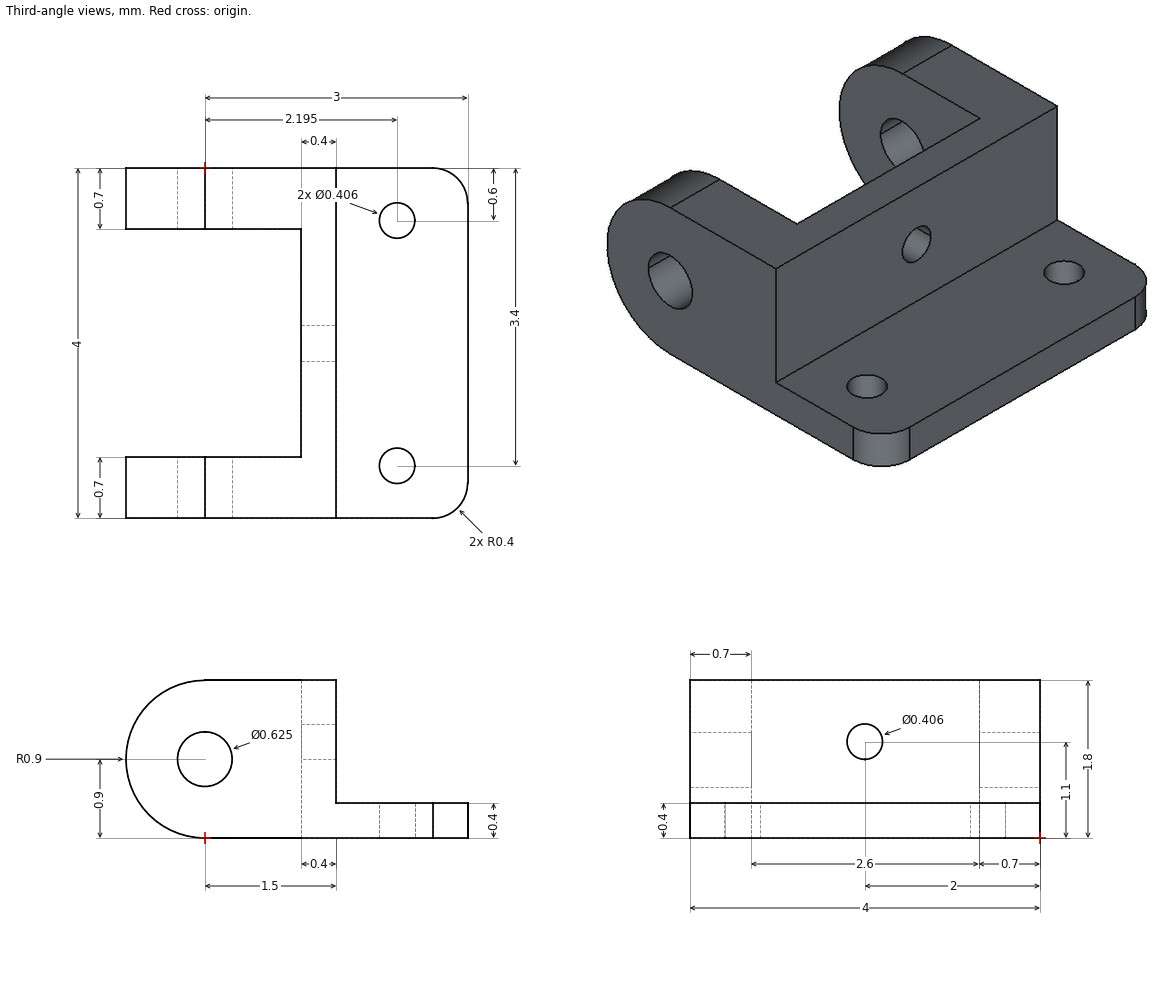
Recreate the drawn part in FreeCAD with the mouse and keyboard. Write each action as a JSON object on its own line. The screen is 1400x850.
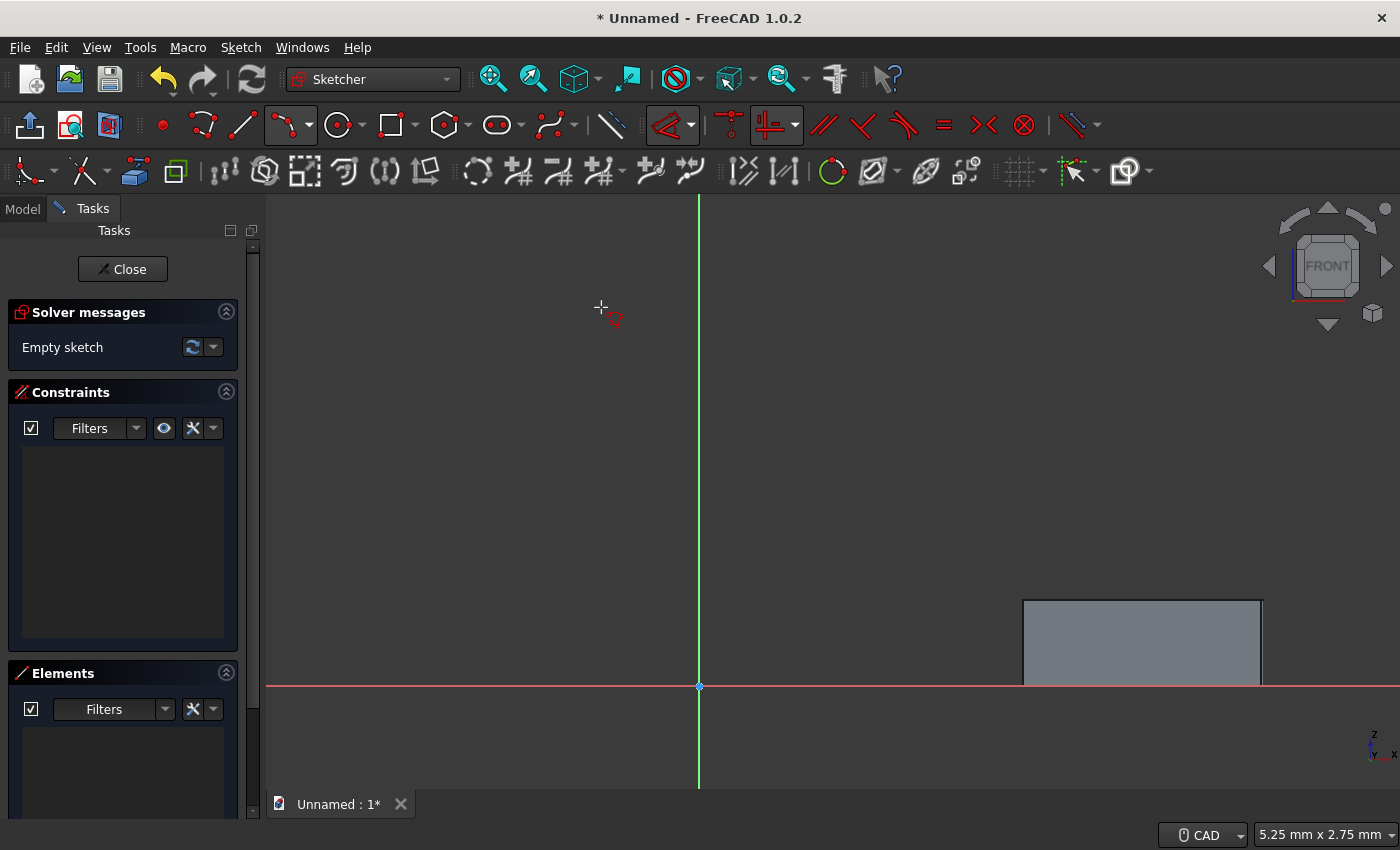
{"action": "left_click", "coordinate": [699, 297]}
{"action": "left_click", "coordinate": [1023, 297]}
{"action": "left_click", "coordinate": [1023, 686]}
{"action": "left_click", "coordinate": [699, 686]}
{"action": "right_click", "coordinate": [699, 686]}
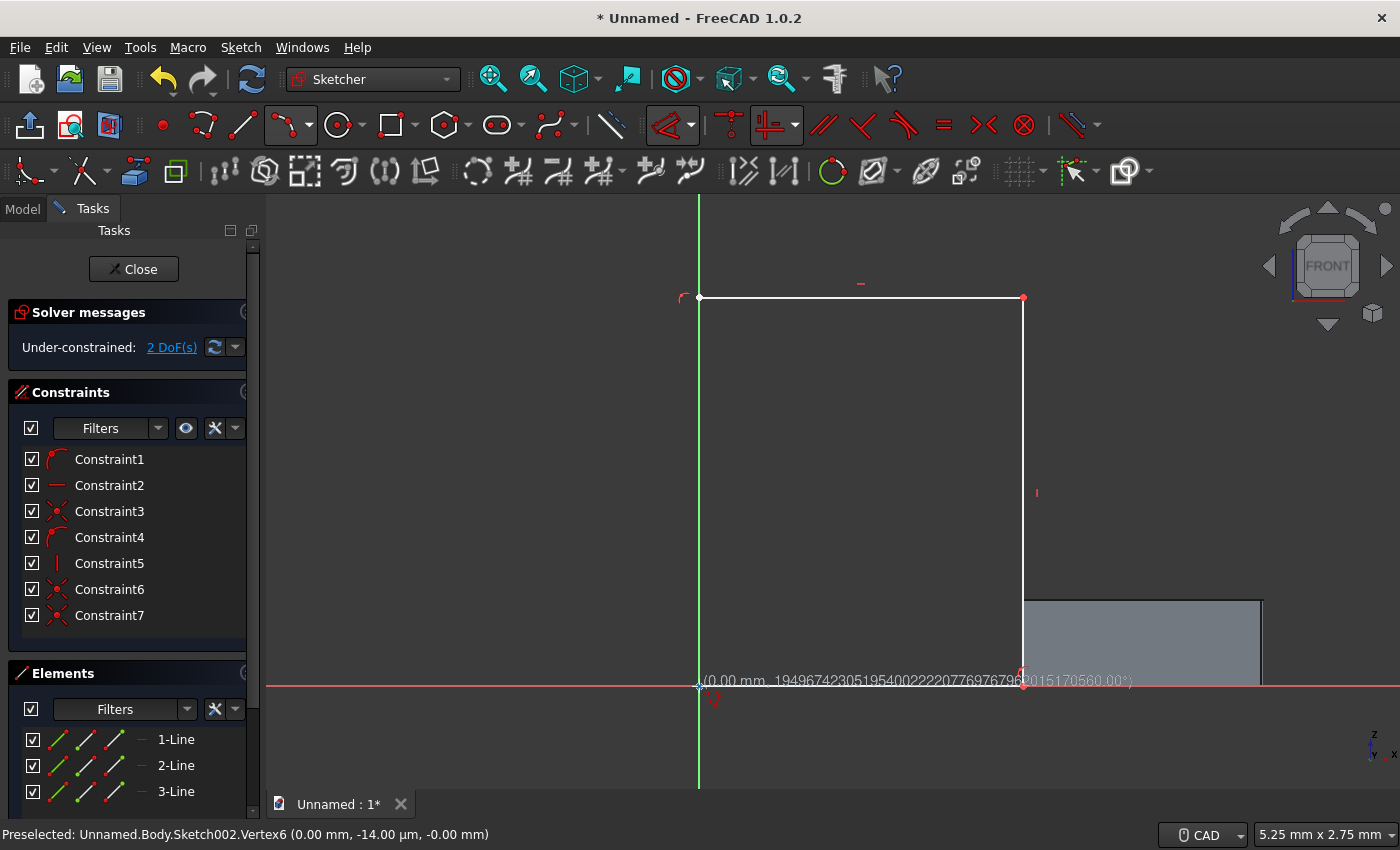
{"action": "left_click", "coordinate": [284, 126]}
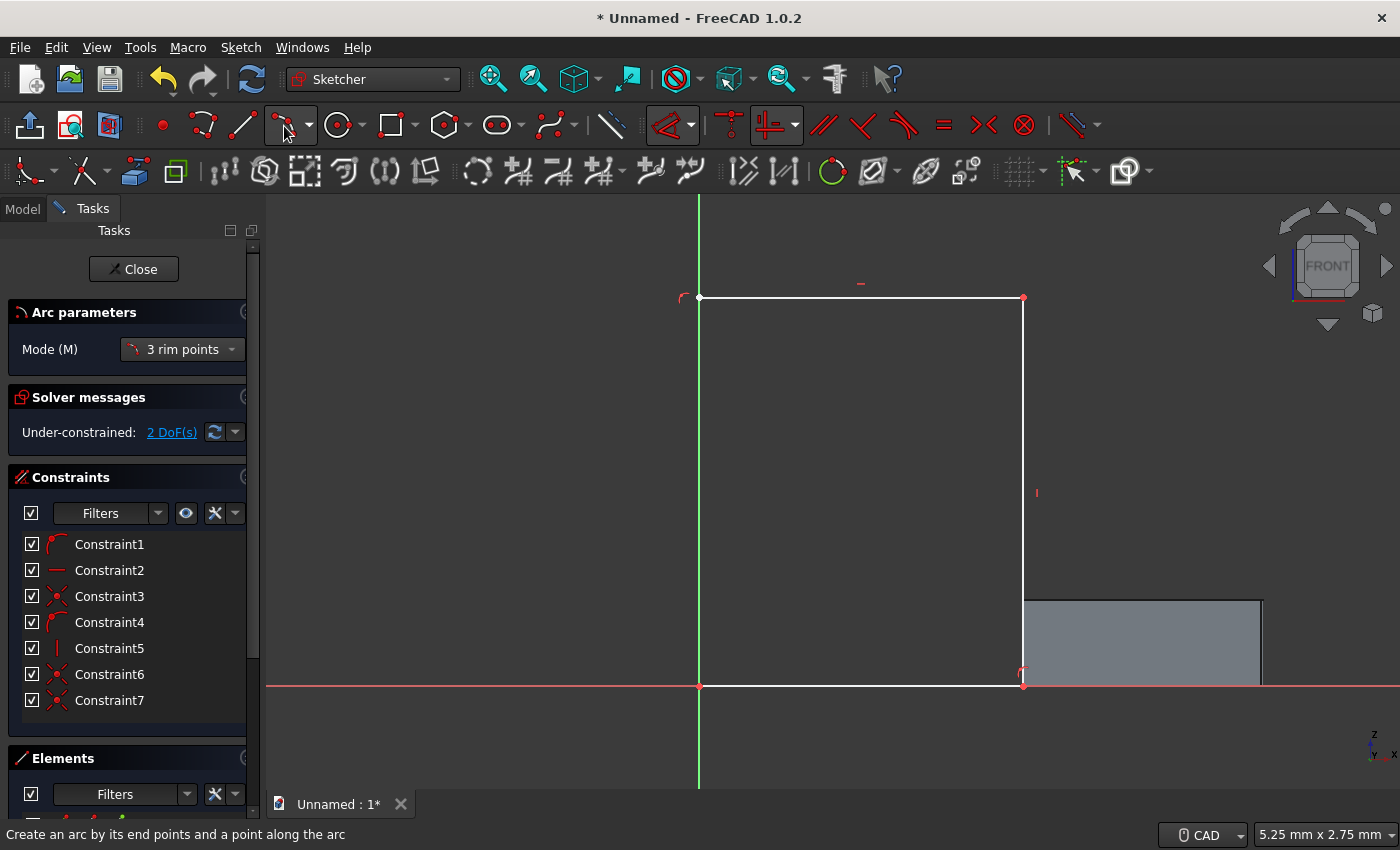
{"action": "left_click", "coordinate": [699, 686]}
{"action": "left_click", "coordinate": [699, 298]}
{"action": "left_click", "coordinate": [505, 492]}
{"action": "key", "text": "Escape"}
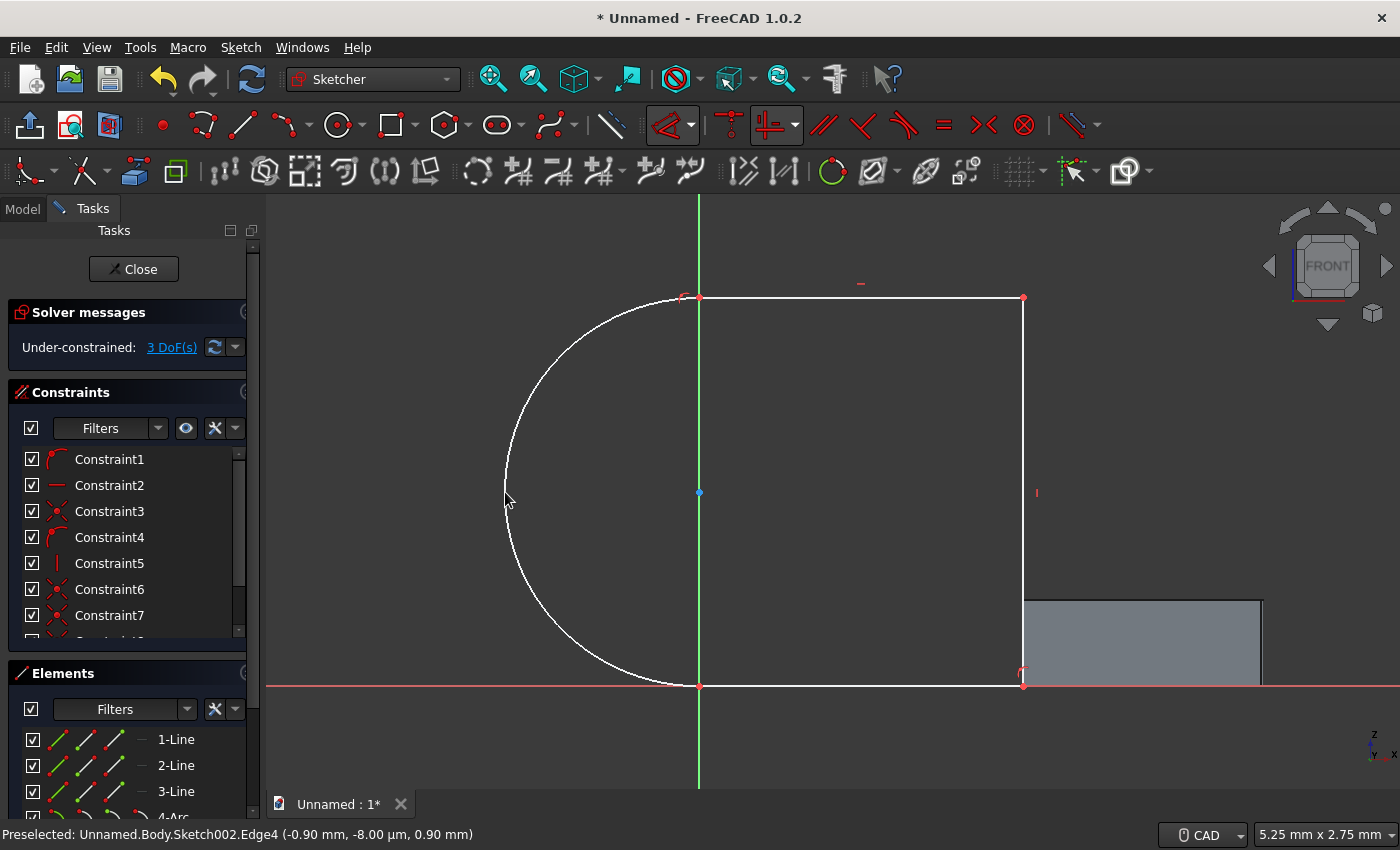
{"action": "left_click", "coordinate": [796, 298]}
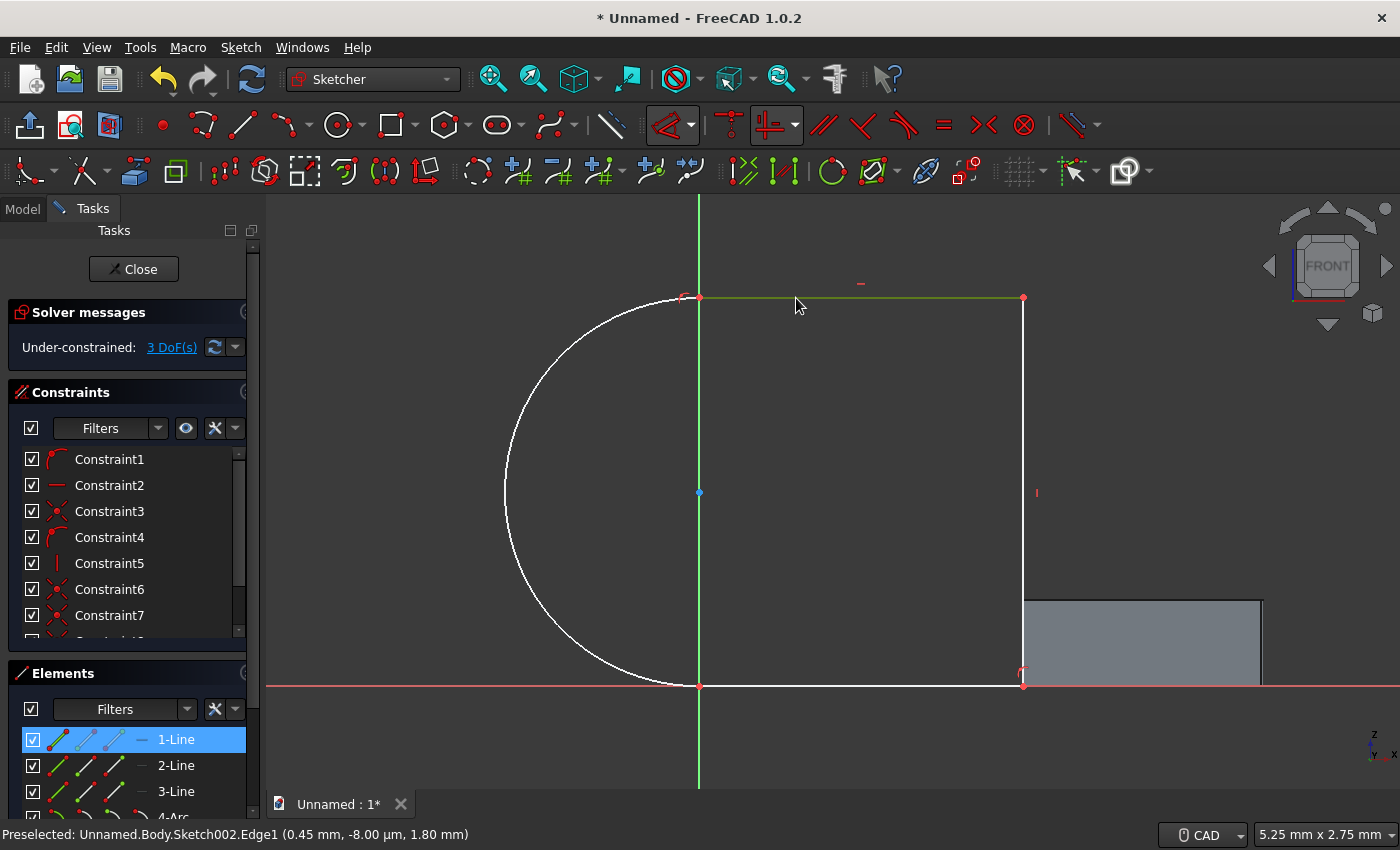
{"action": "left_click", "coordinate": [542, 378]}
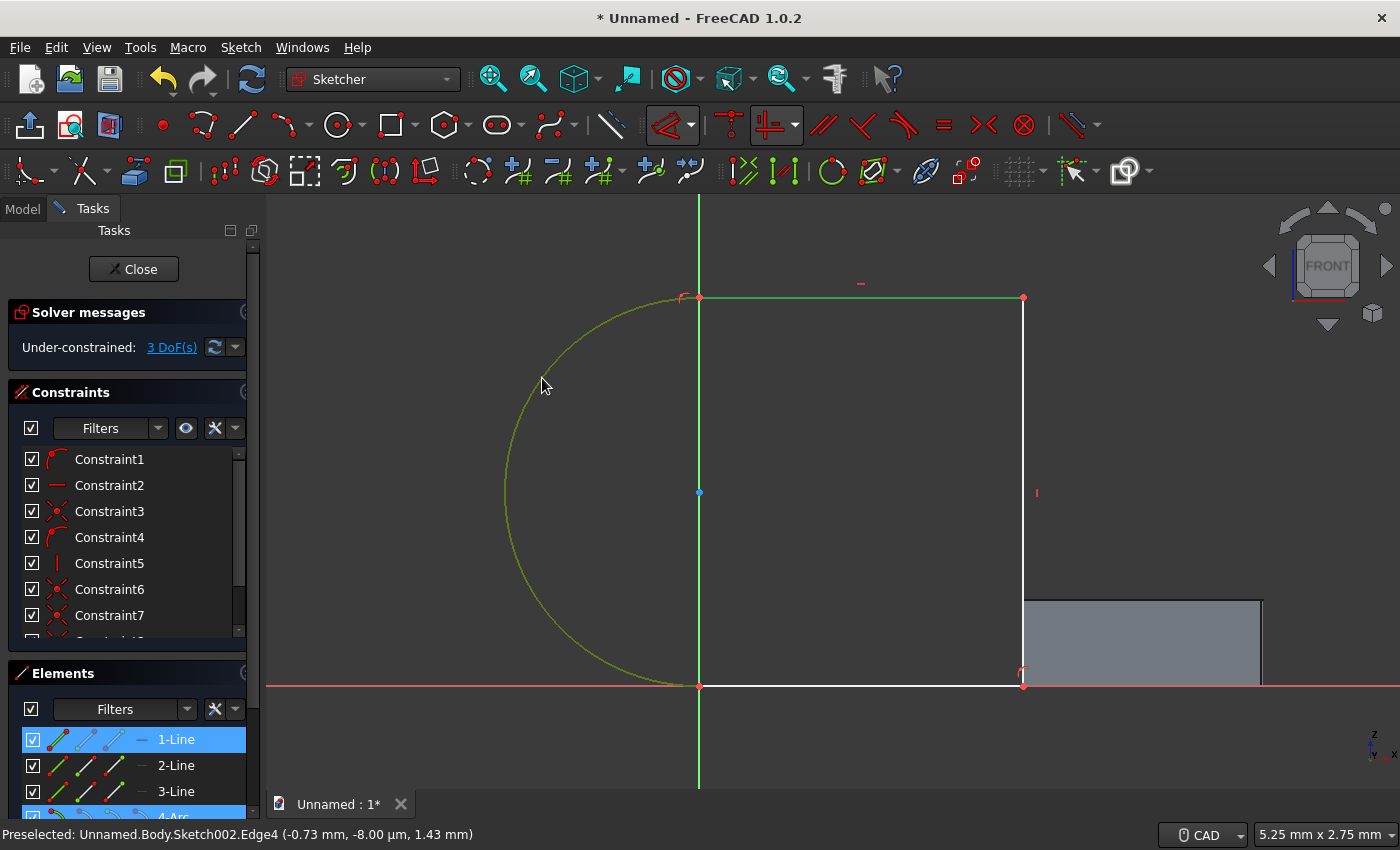
{"action": "key", "text": "t"}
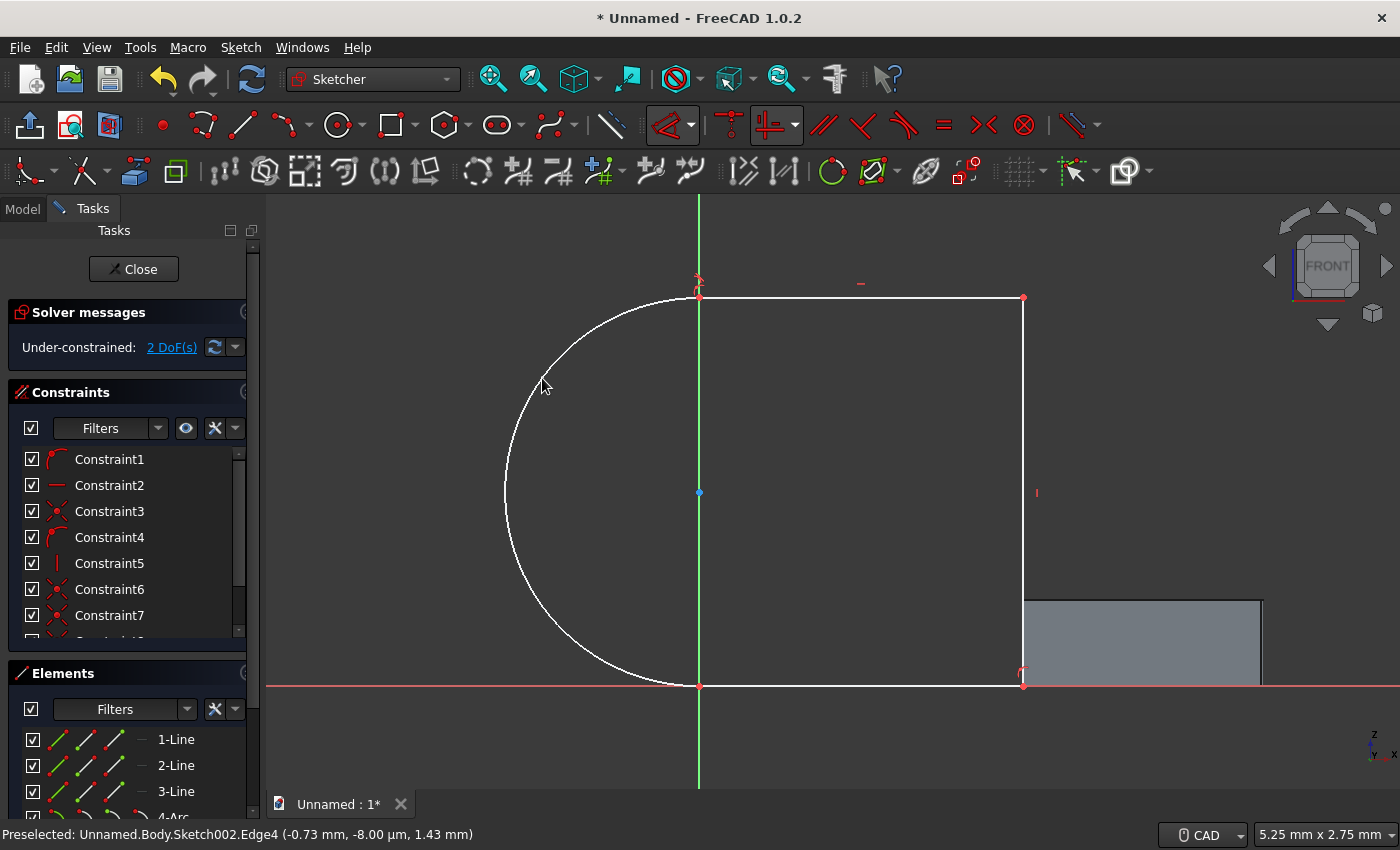
{"action": "left_click", "coordinate": [666, 126]}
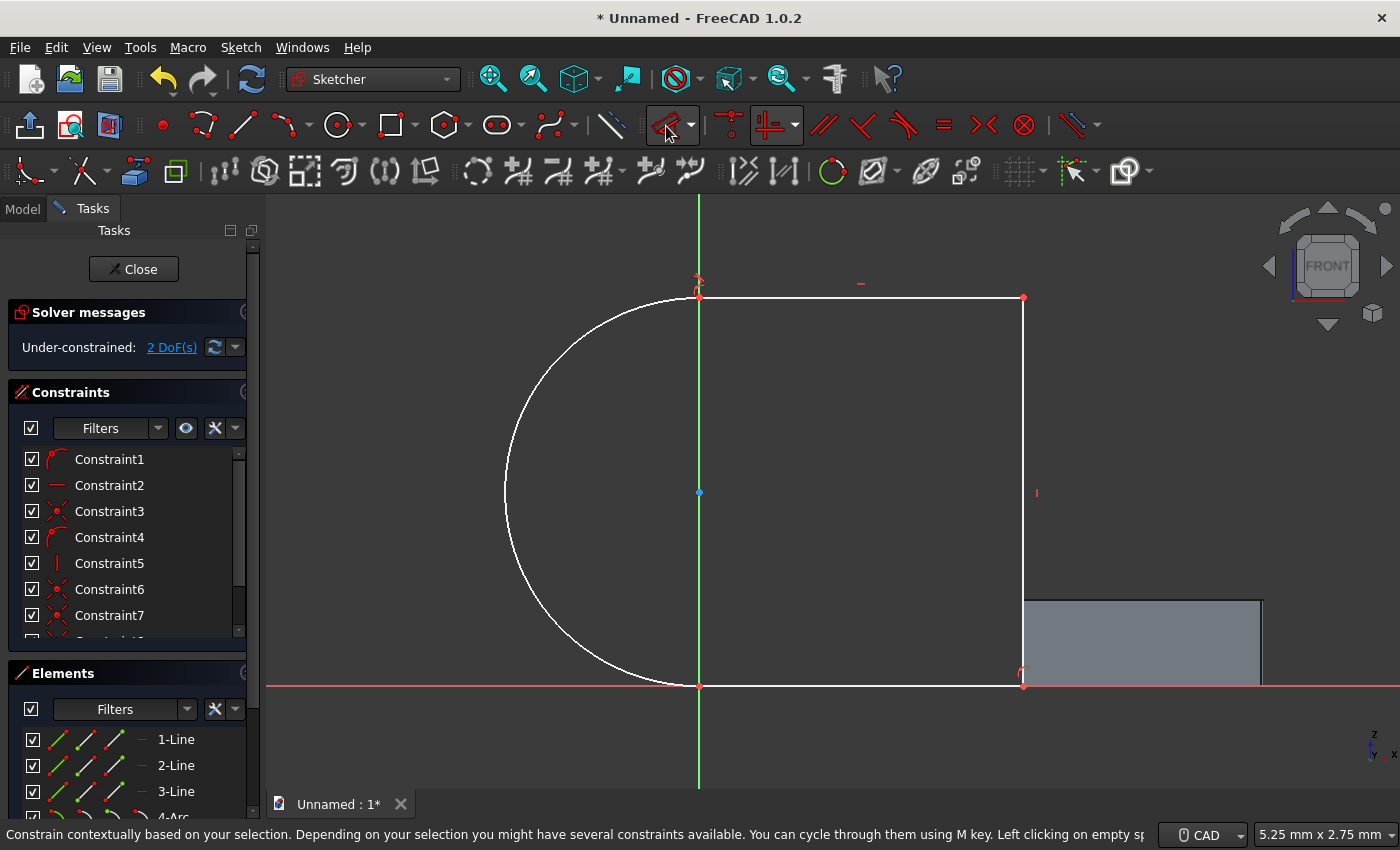
{"action": "left_click", "coordinate": [542, 378]}
{"action": "left_click", "coordinate": [516, 359]}